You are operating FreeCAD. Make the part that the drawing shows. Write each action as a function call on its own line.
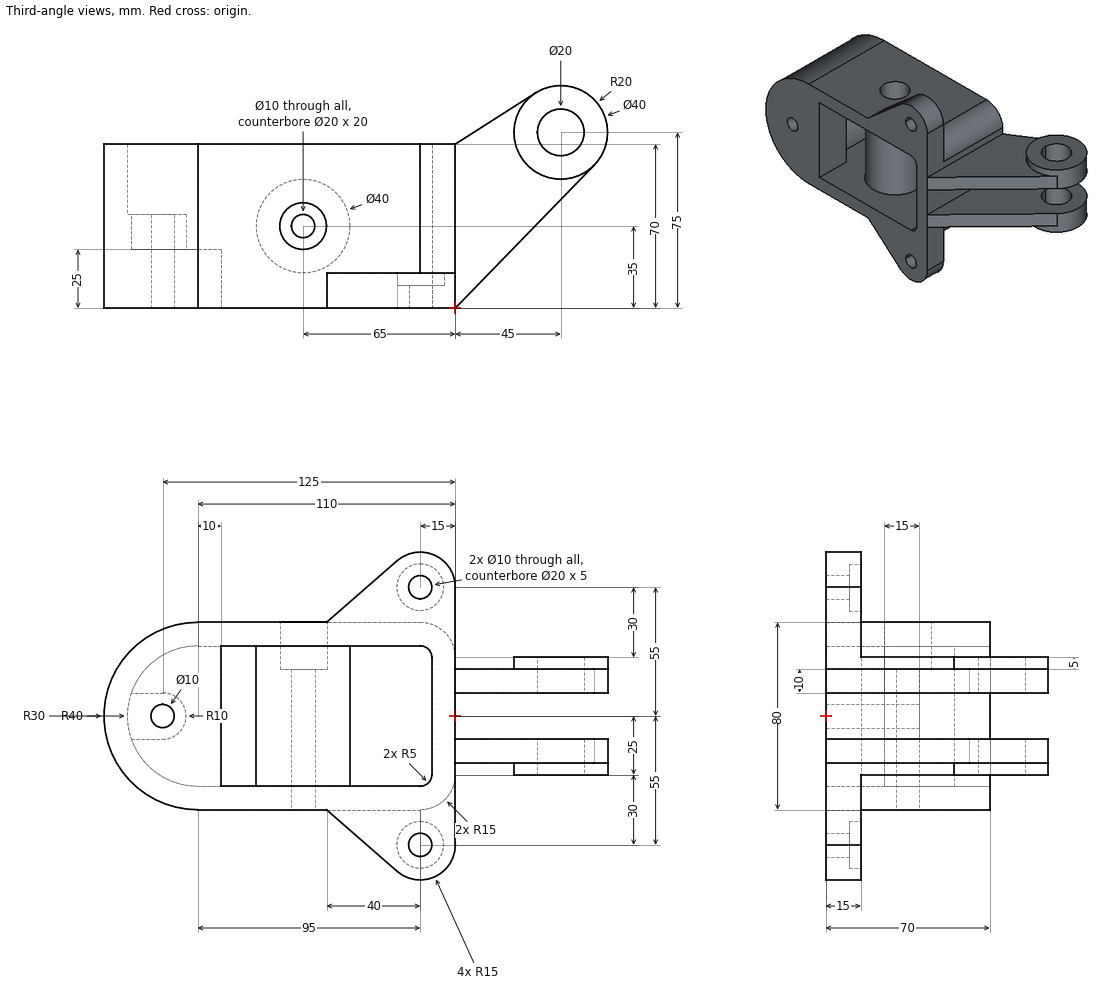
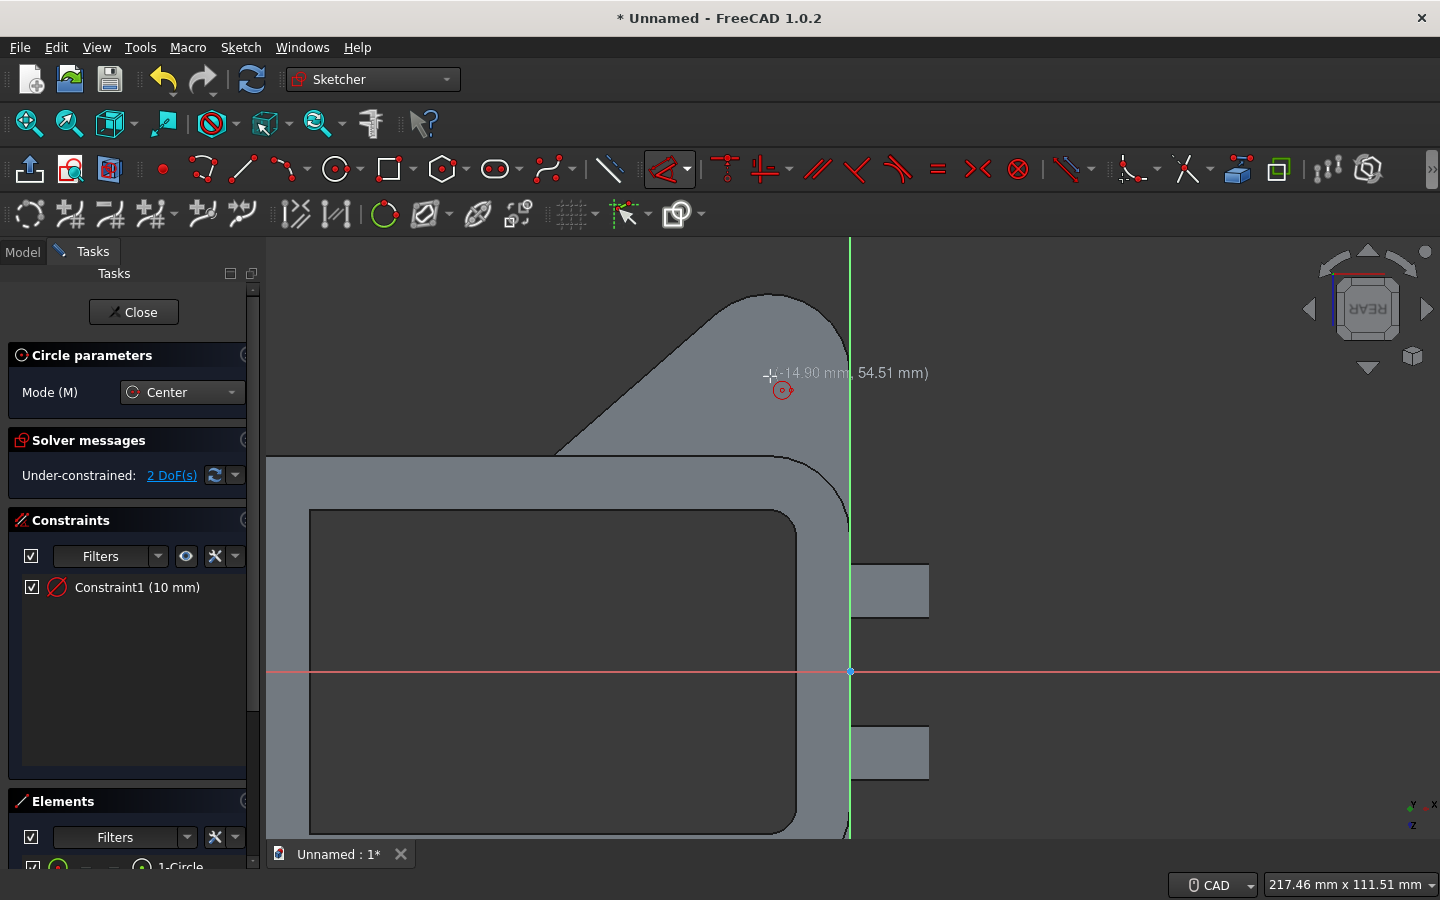
click(769, 375)
move(788, 356)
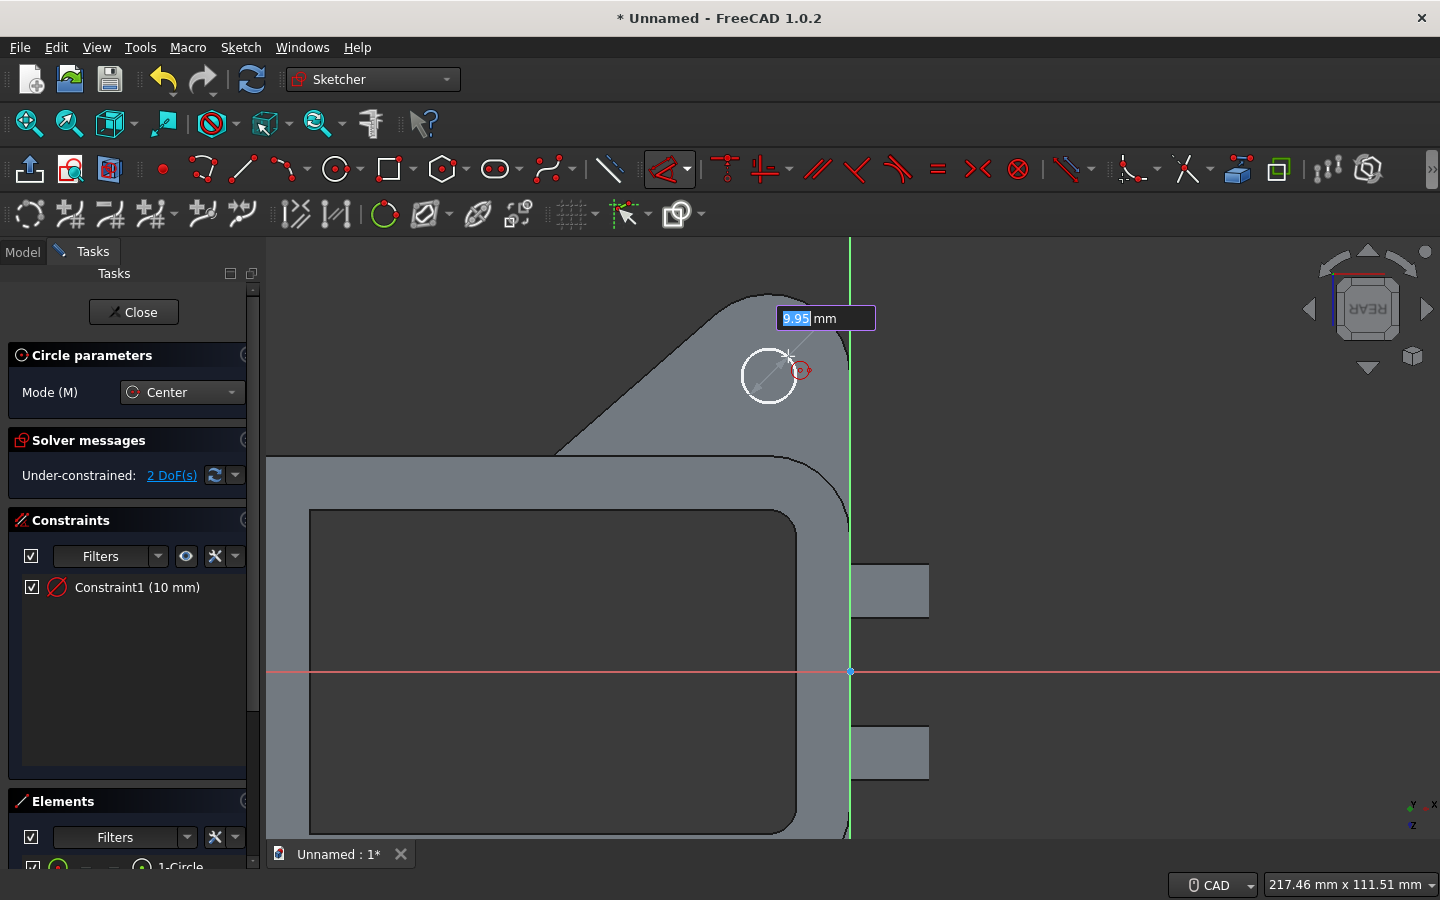
text(10)
key(Return)
key(Escape)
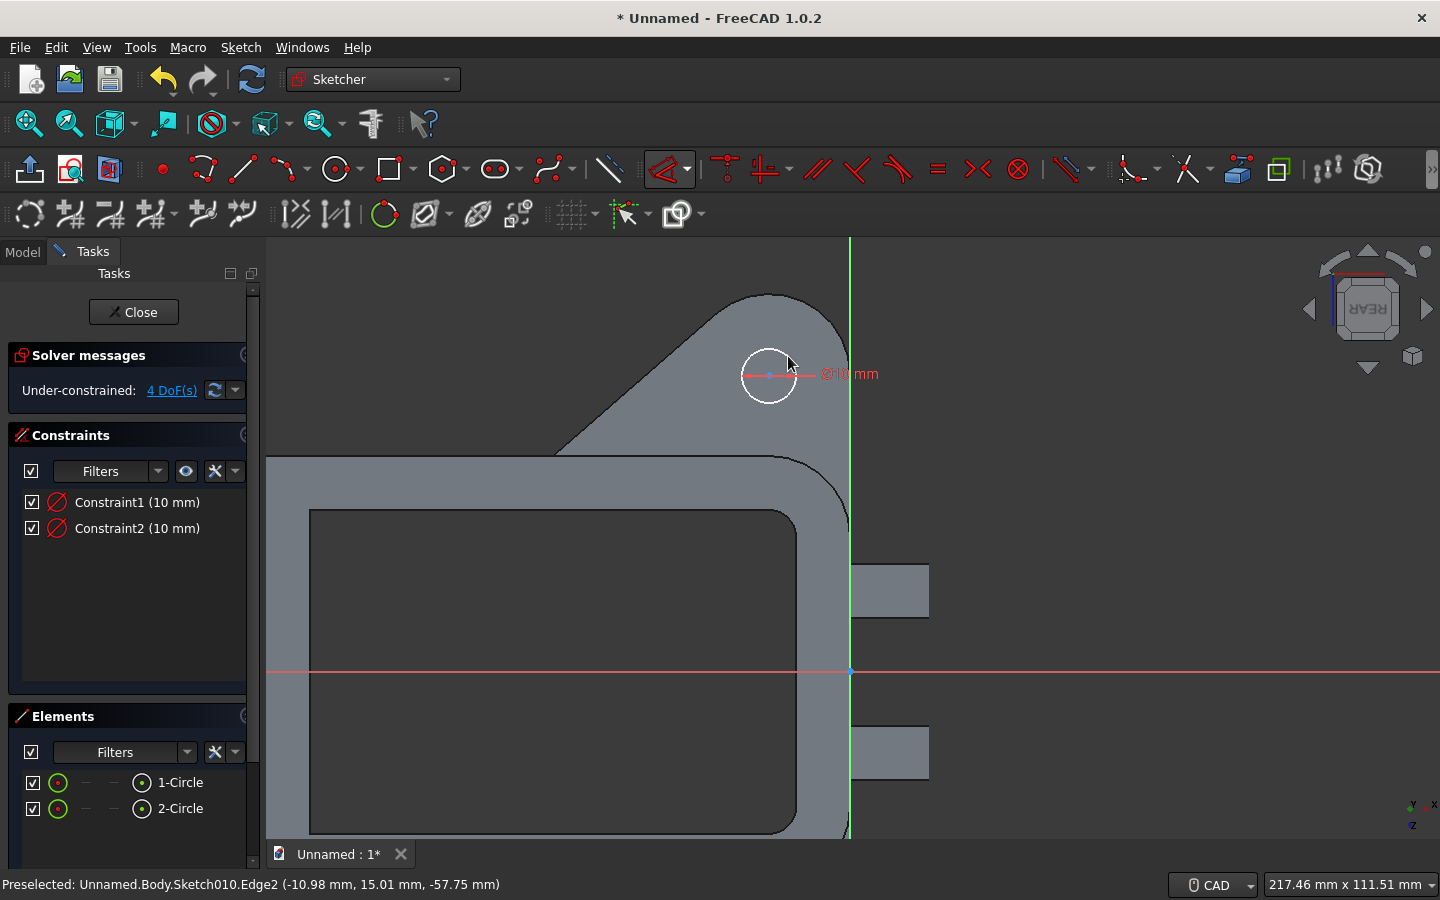
scroll(770, 375, down, 3)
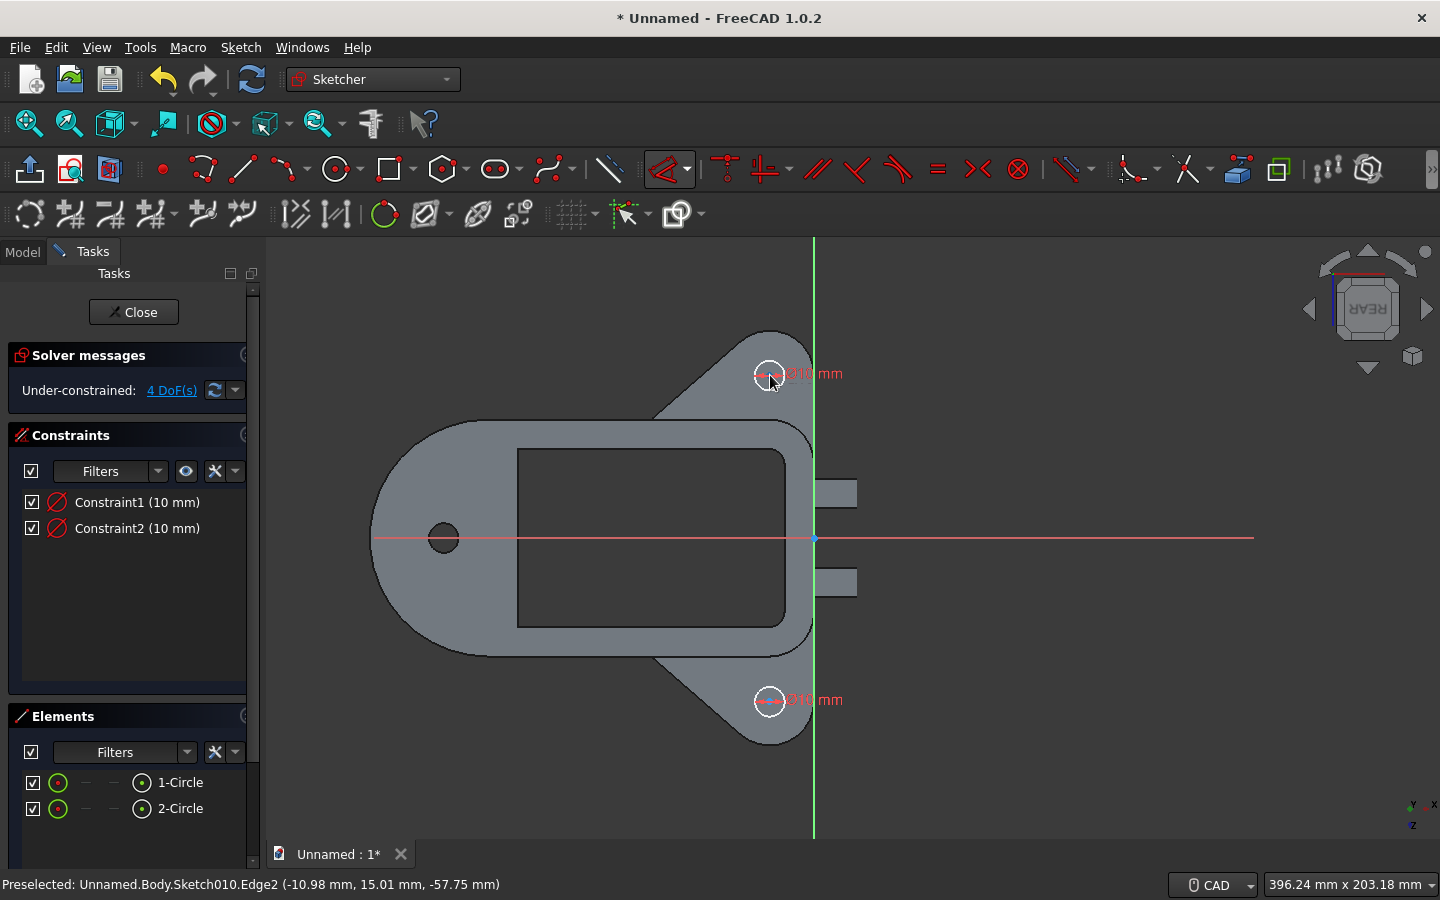
click(770, 702)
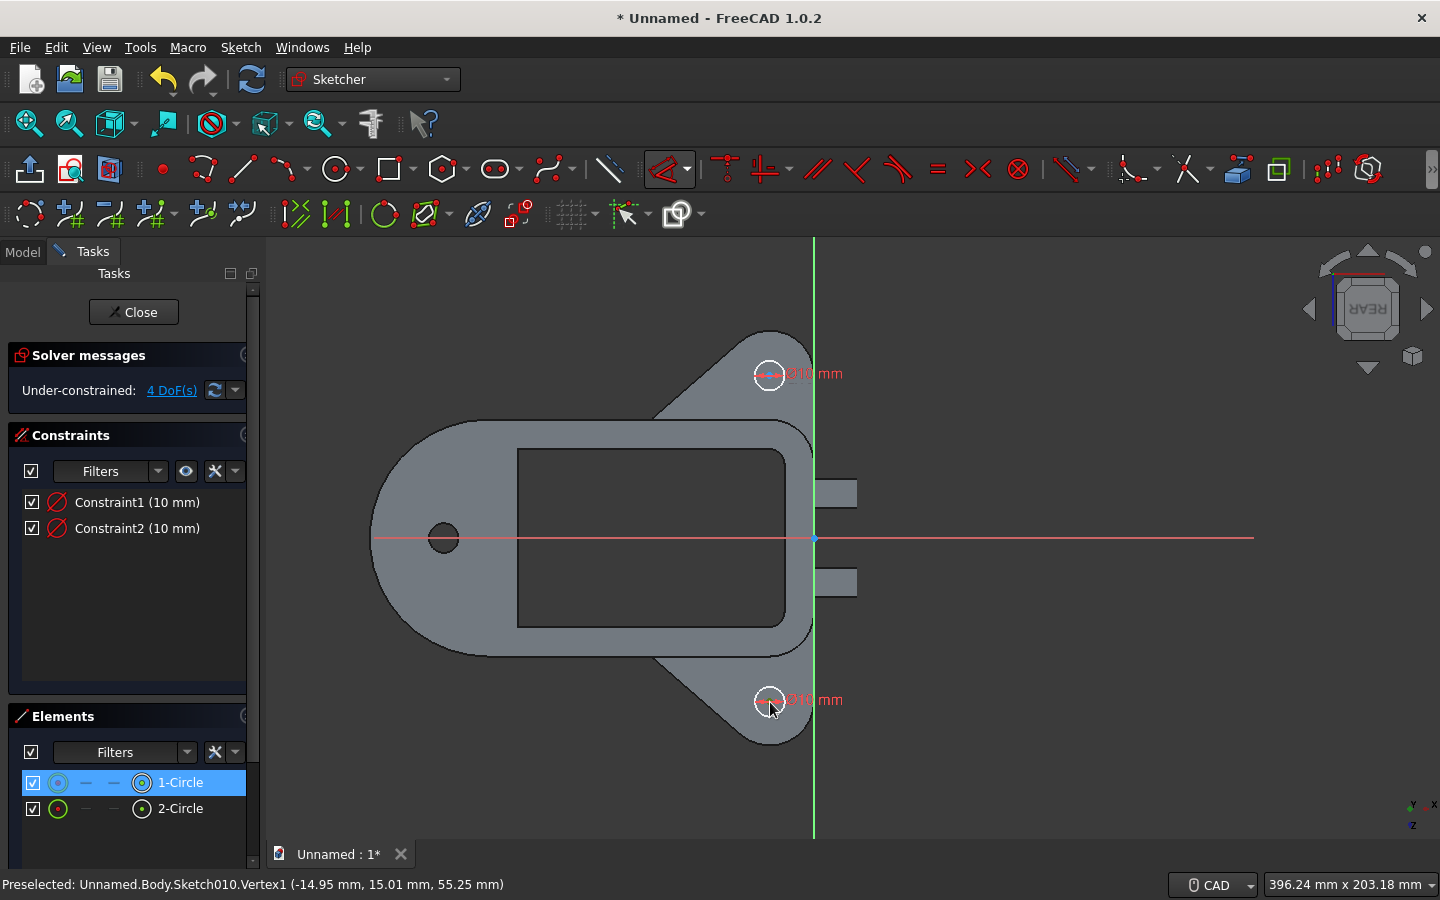
click(770, 376)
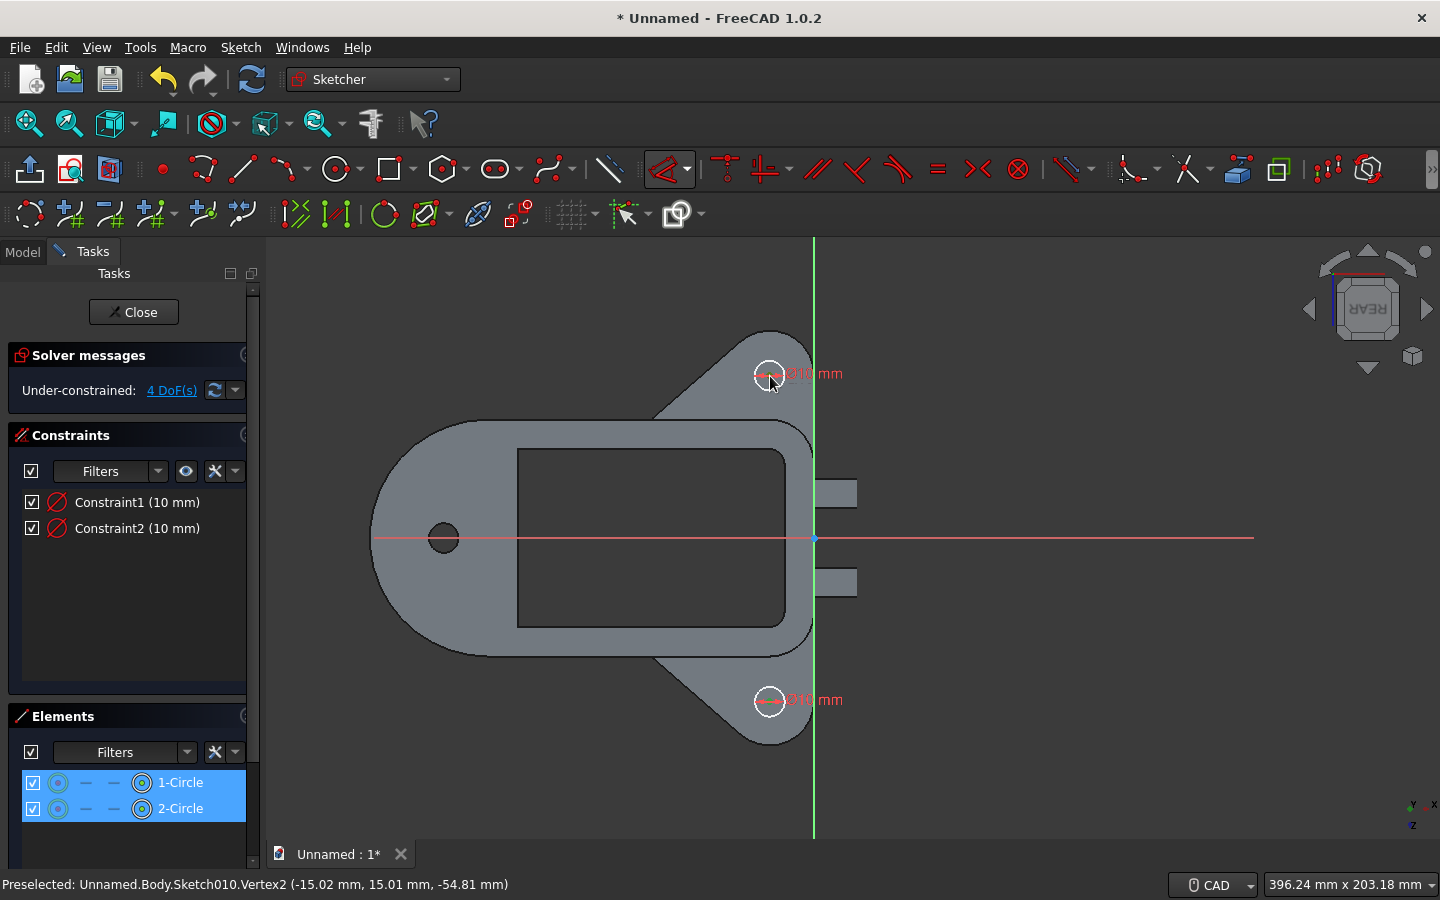
key(v)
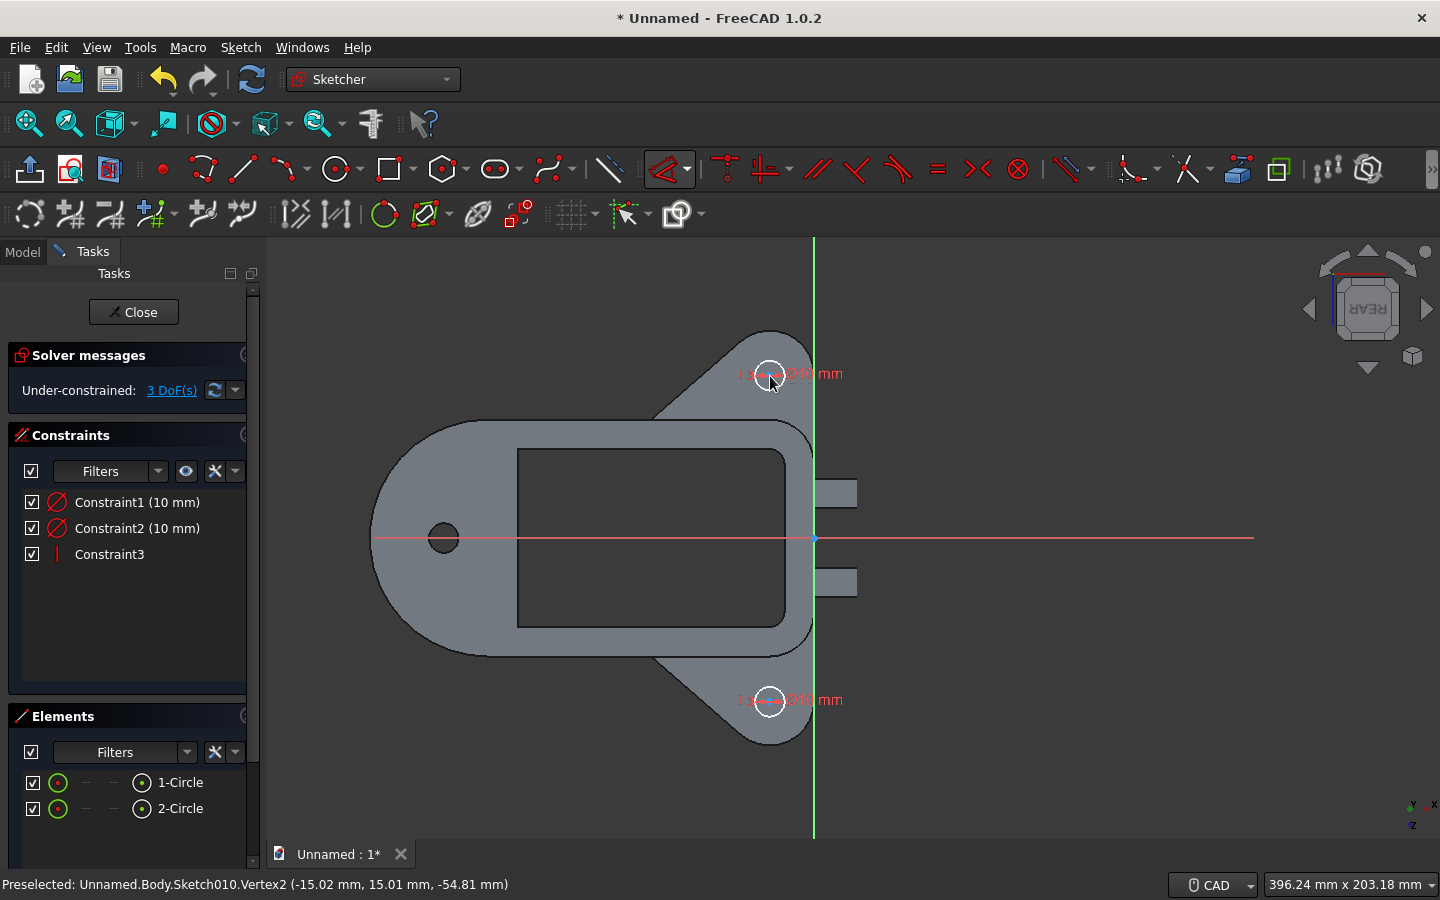
click(770, 702)